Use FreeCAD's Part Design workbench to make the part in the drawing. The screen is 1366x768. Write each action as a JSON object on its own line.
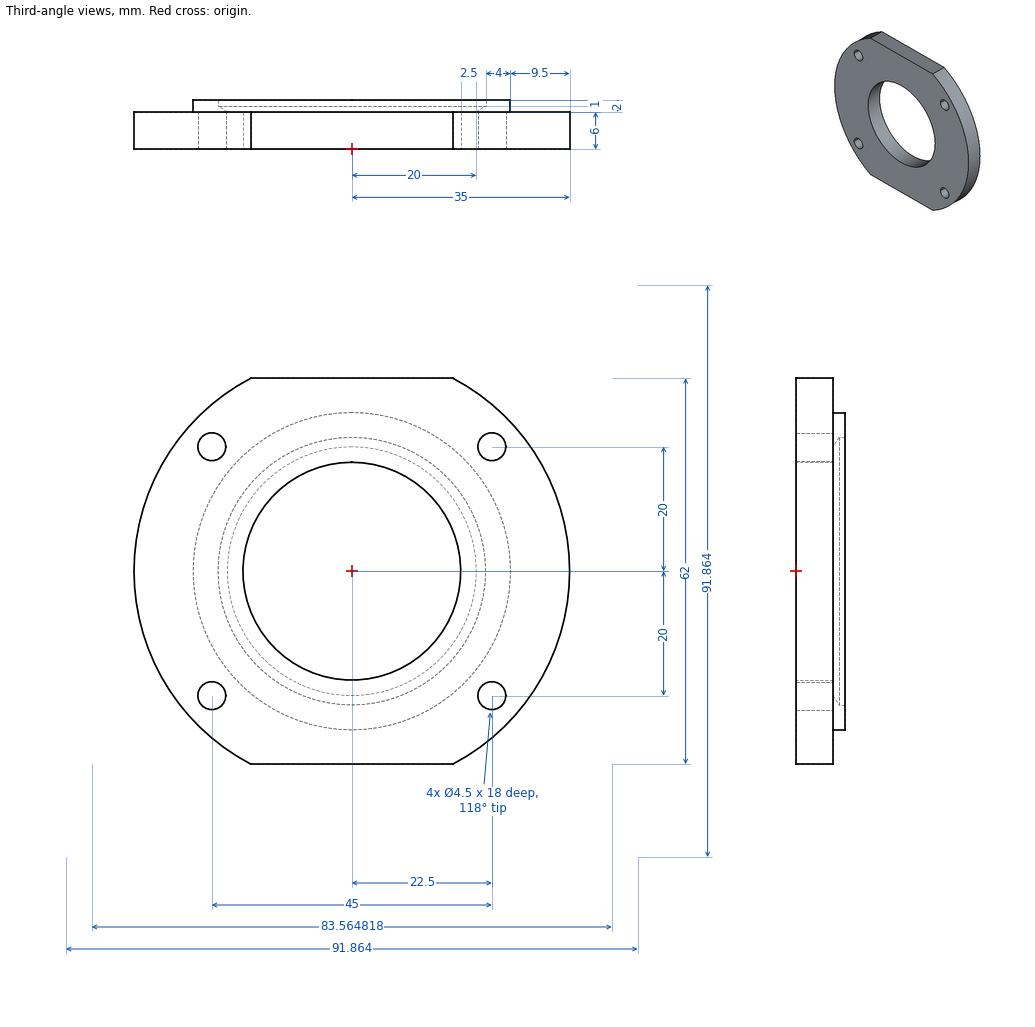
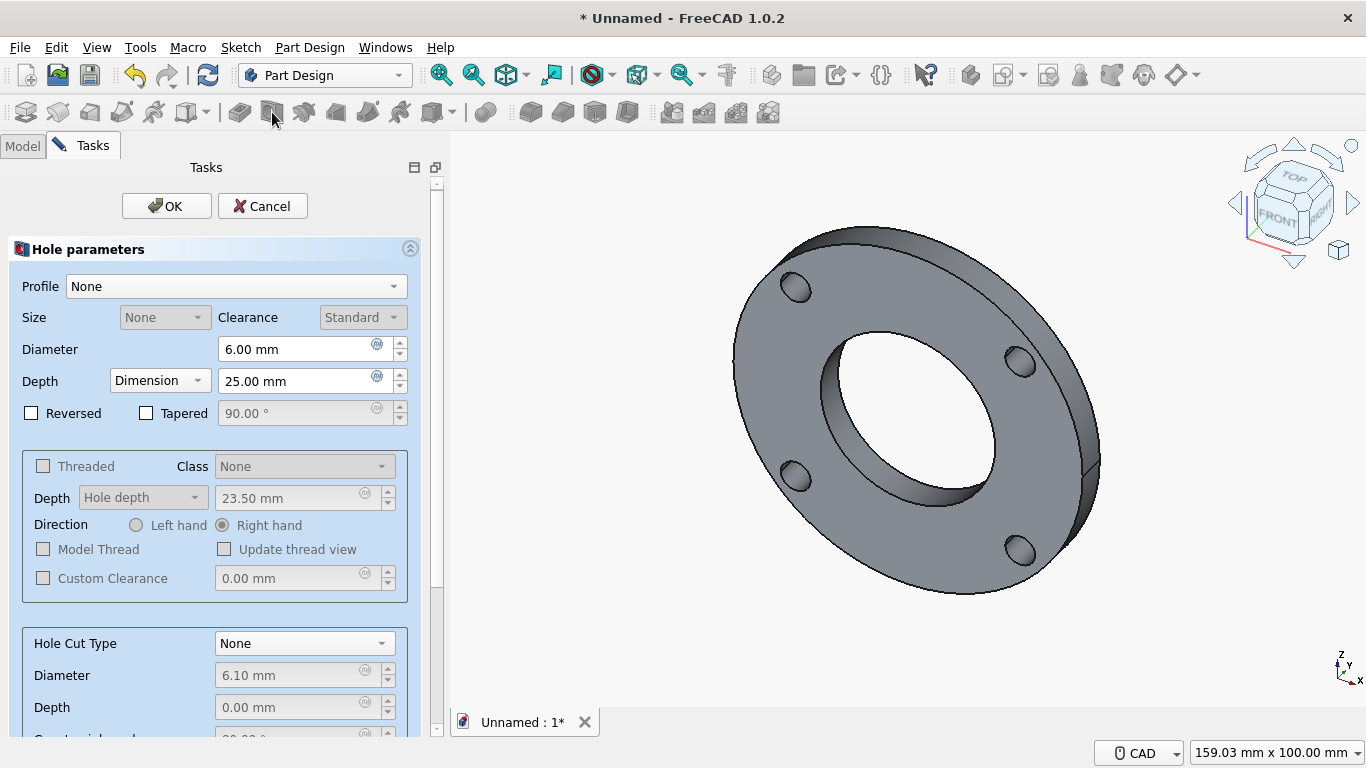
{"action": "triple_click", "coordinate": [305, 349]}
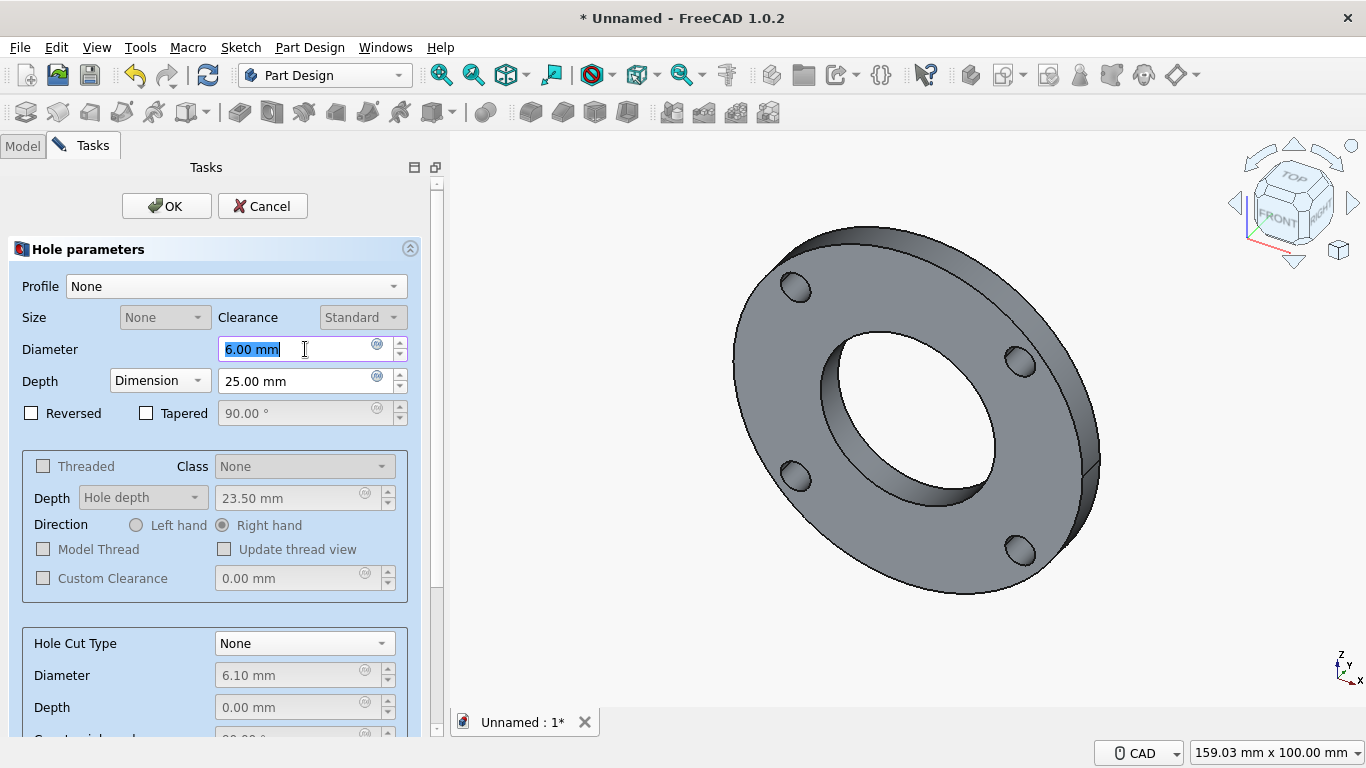
{"action": "type", "text": "4.5"}
{"action": "key", "text": "Tab"}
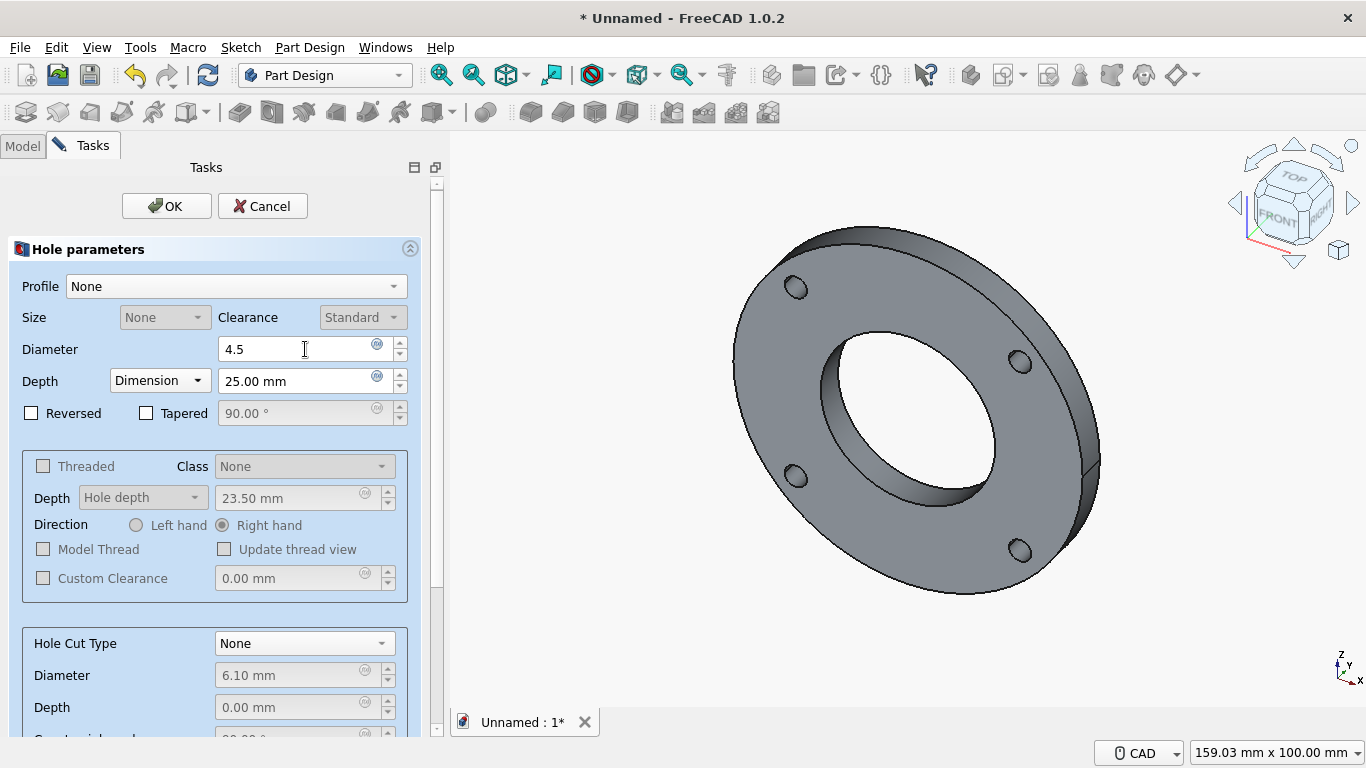
{"action": "triple_click", "coordinate": [305, 381]}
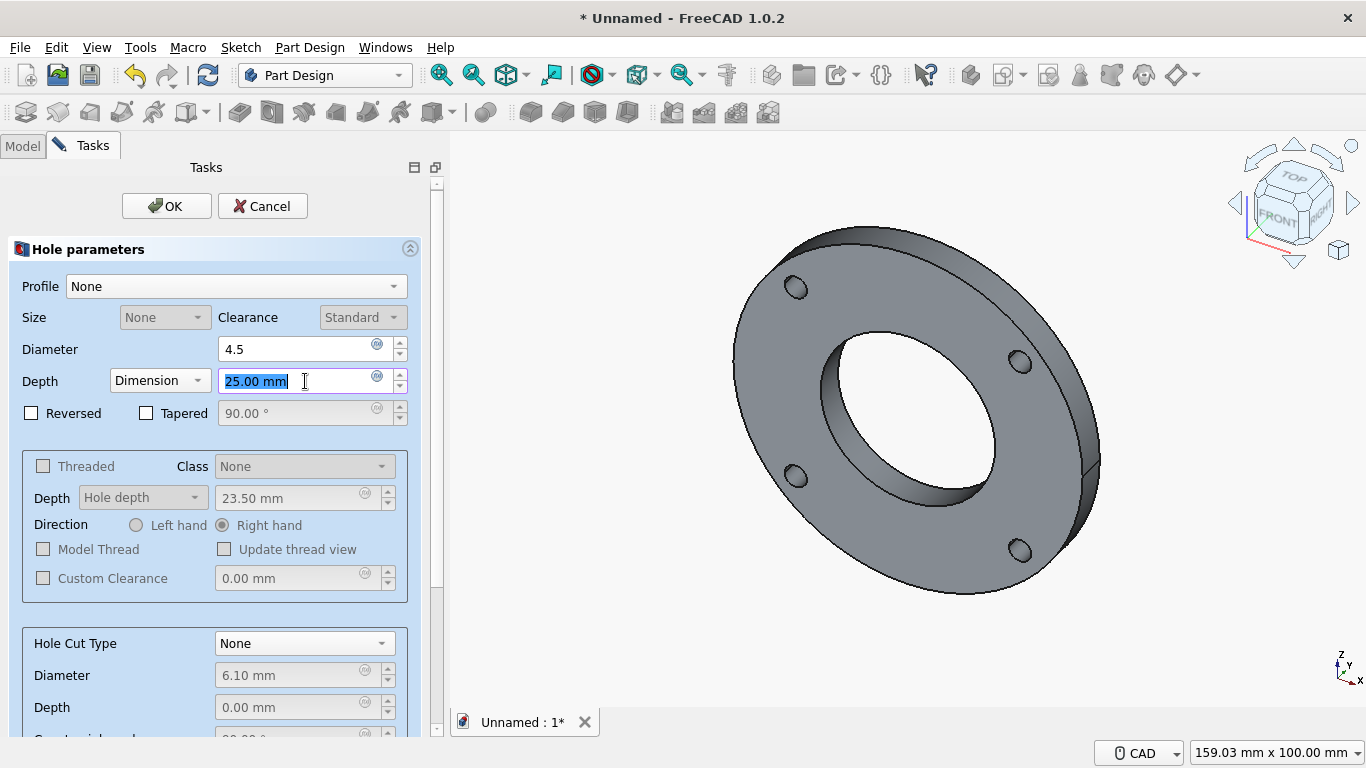
{"action": "type", "text": "18"}
{"action": "key", "text": "Tab"}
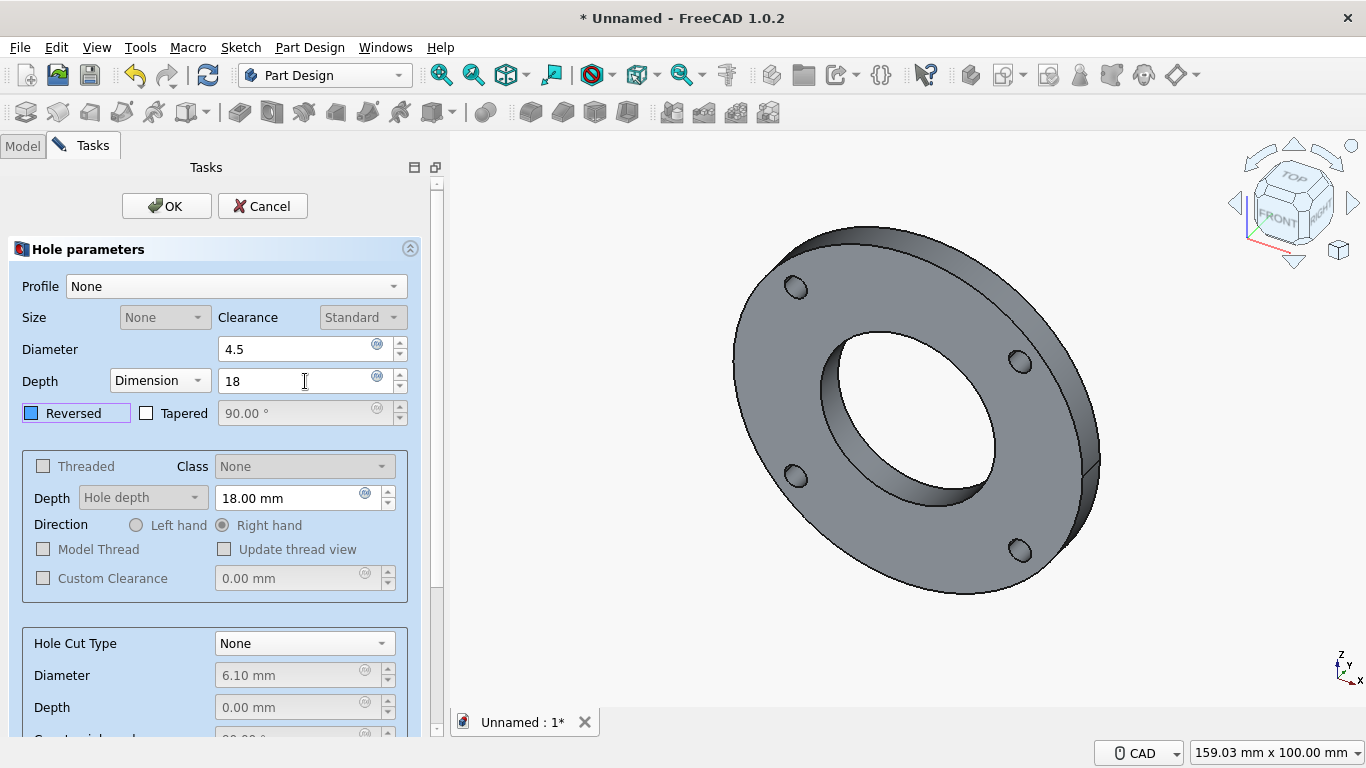
{"action": "left_click", "coordinate": [167, 206]}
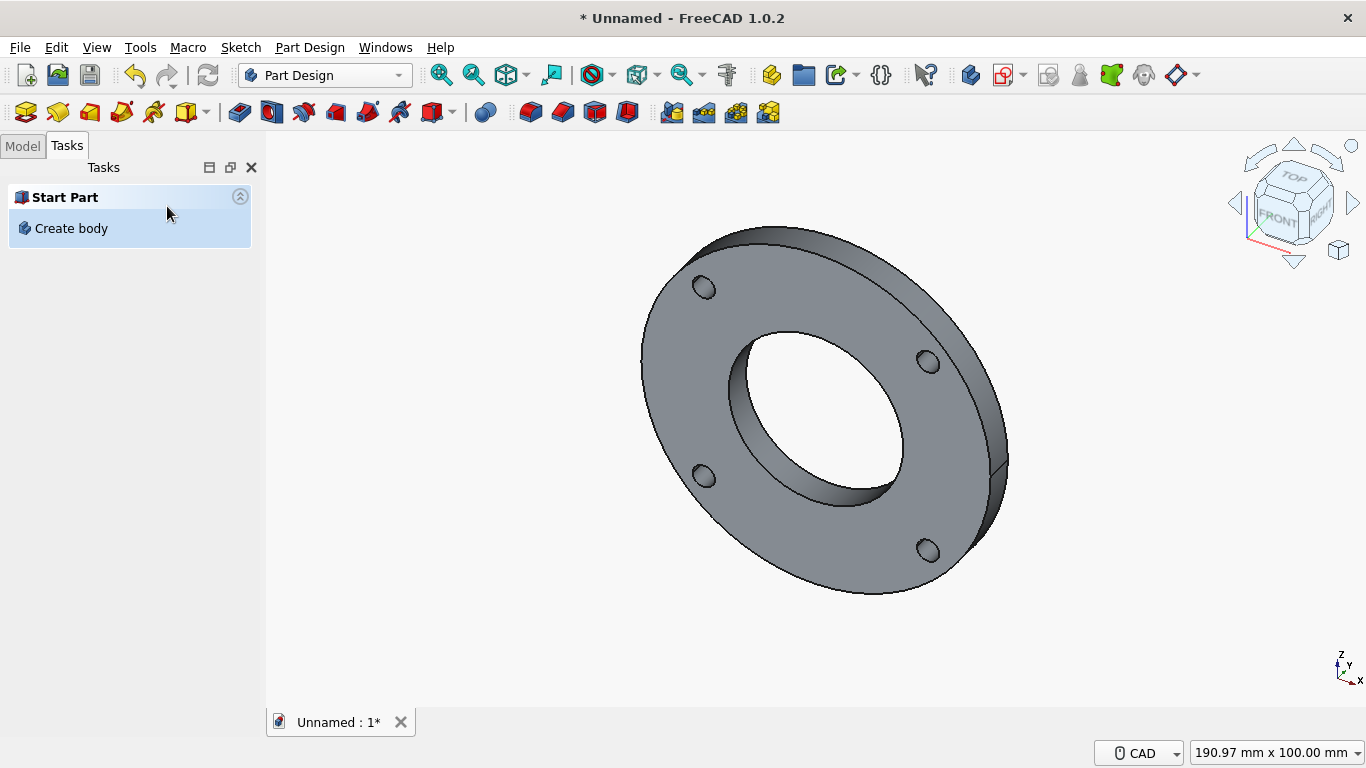
{"action": "left_click", "coordinate": [1004, 76]}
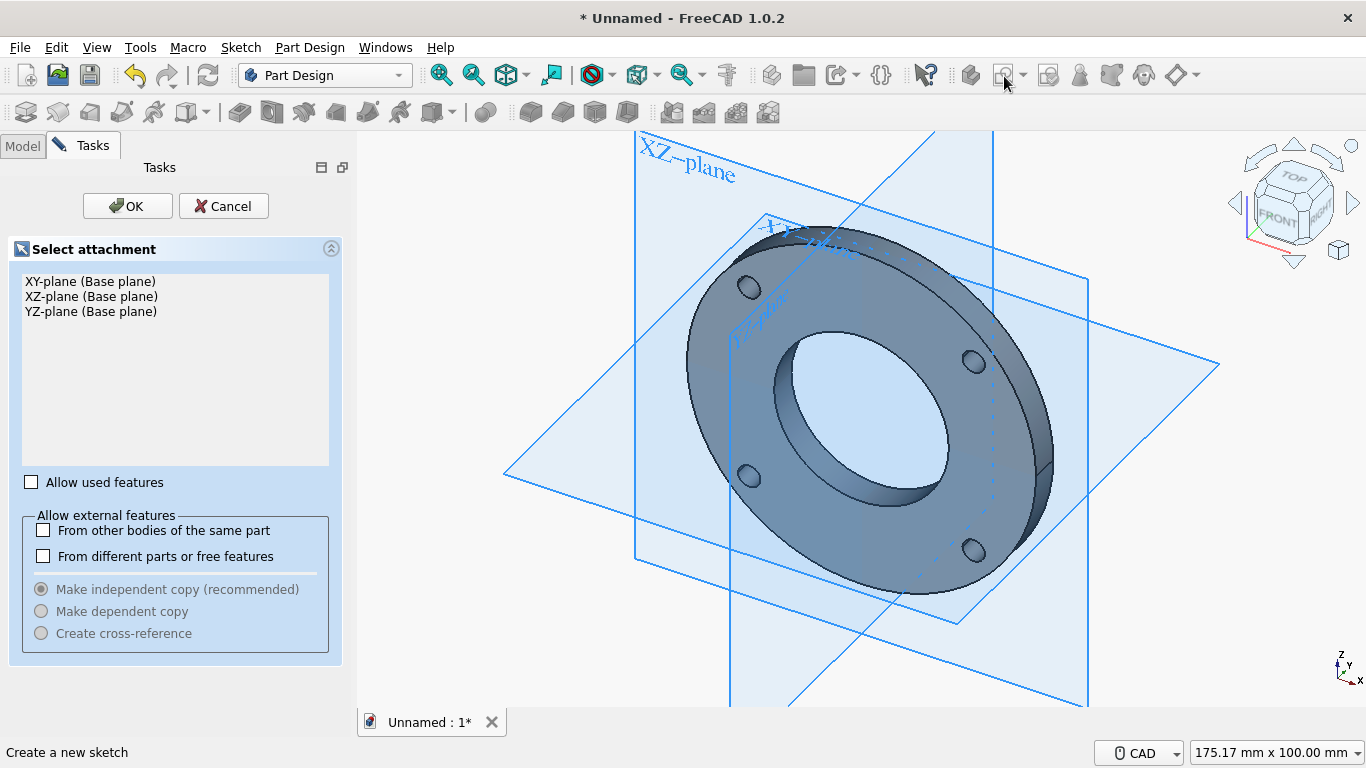
{"action": "left_click", "coordinate": [82, 296]}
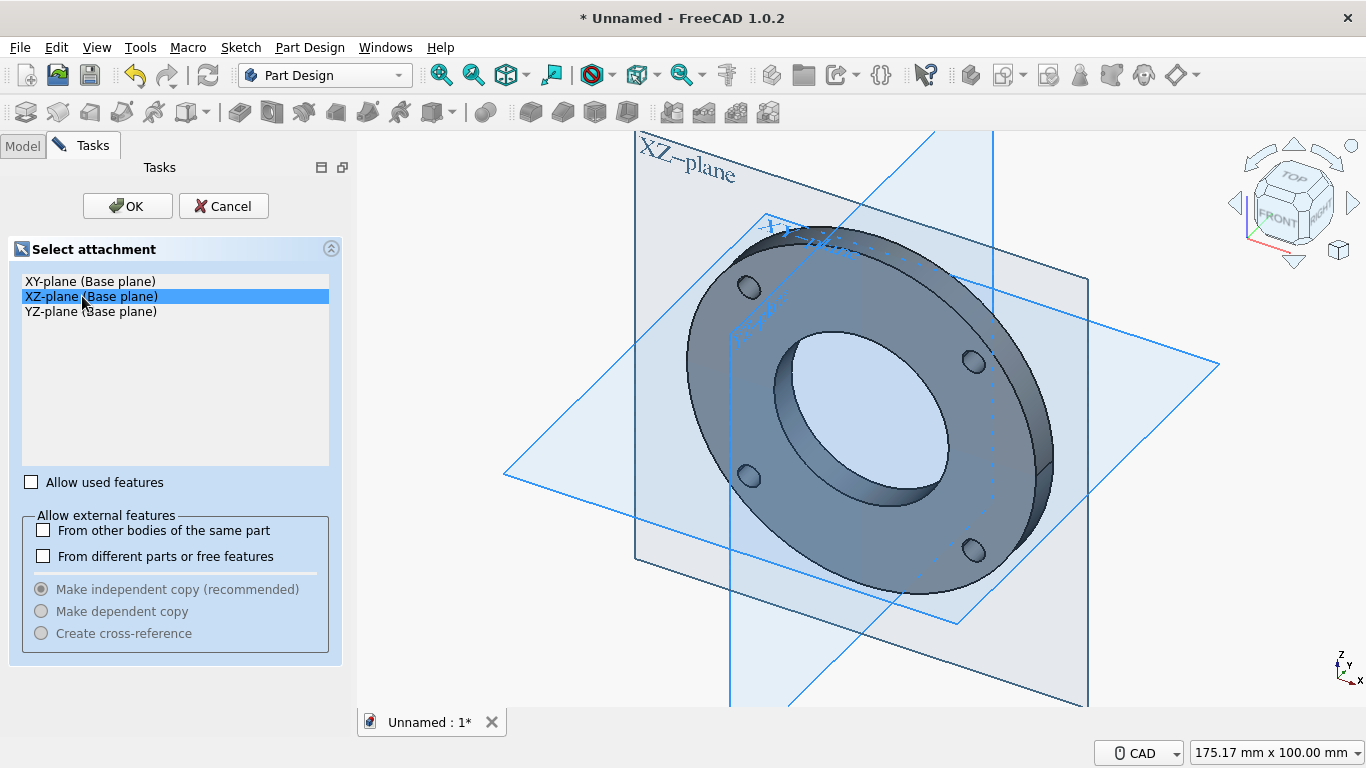
{"action": "left_click", "coordinate": [128, 206]}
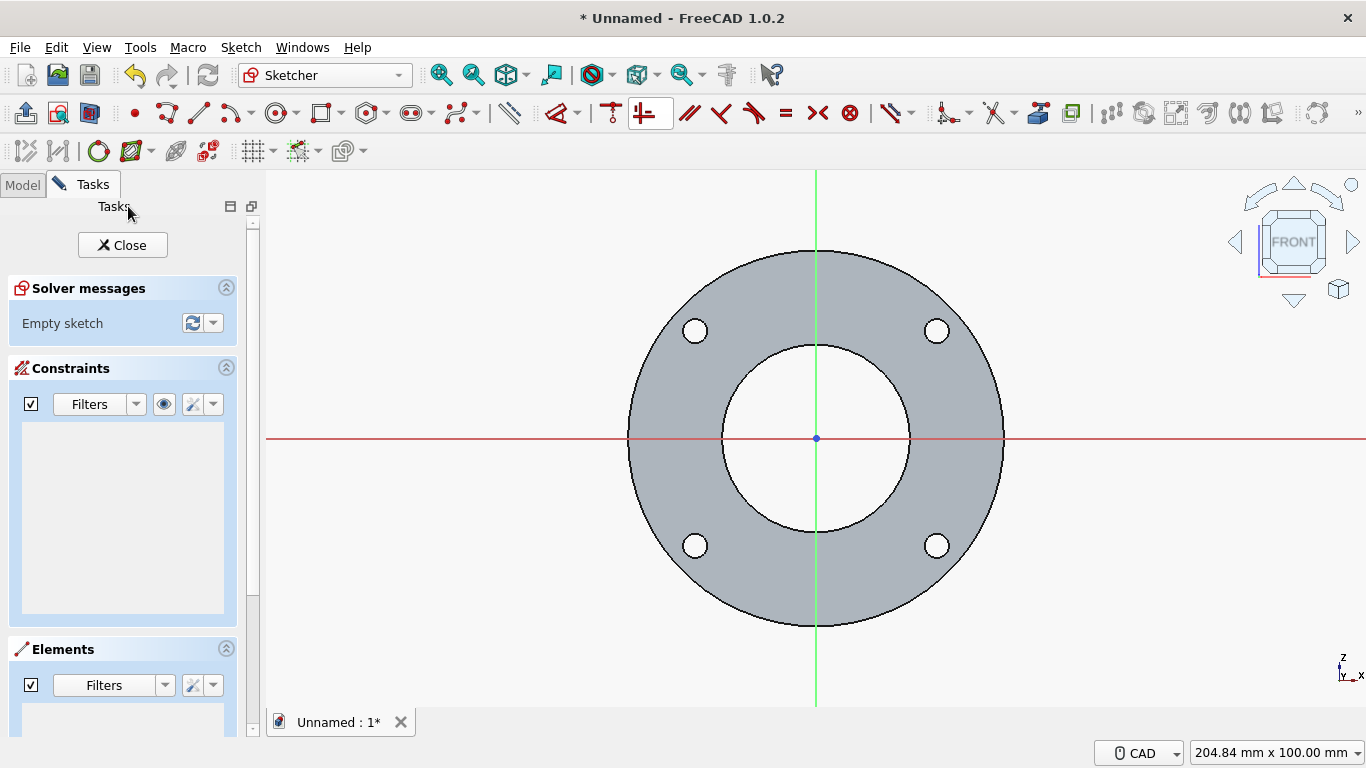
{"action": "scroll", "coordinate": [608, 439], "scroll_direction": "down", "scroll_amount": 2}